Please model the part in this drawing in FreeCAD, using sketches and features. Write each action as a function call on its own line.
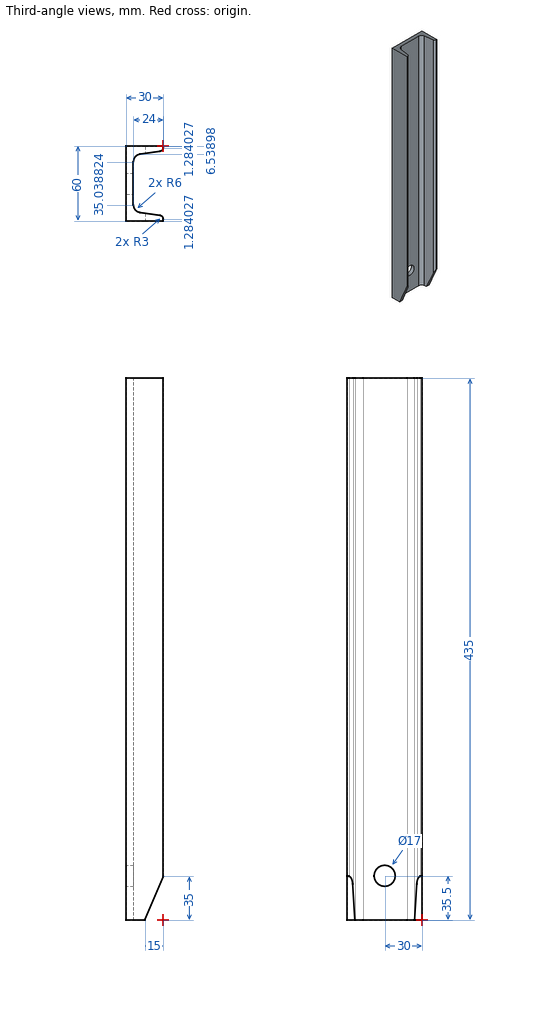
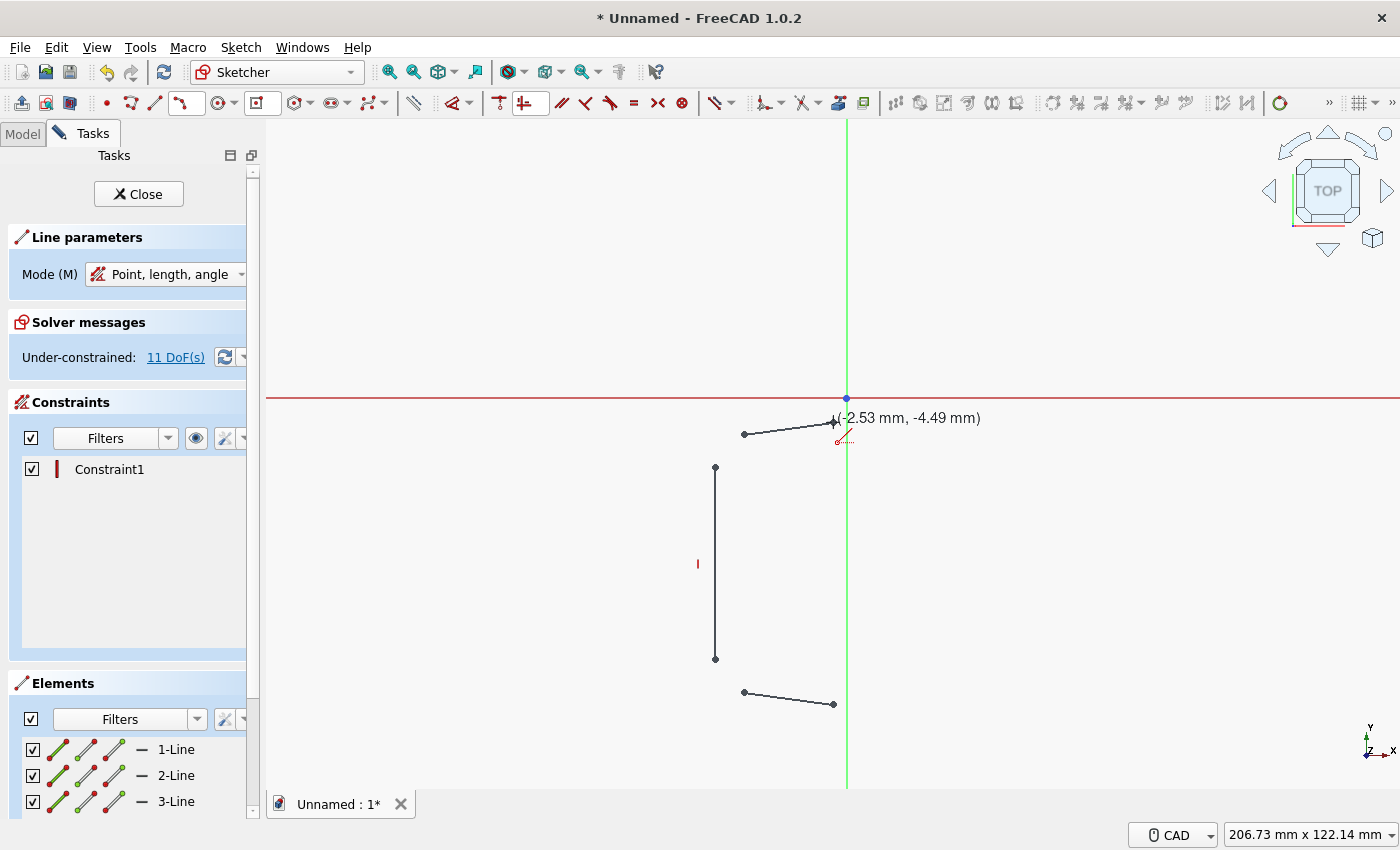
click(132, 104)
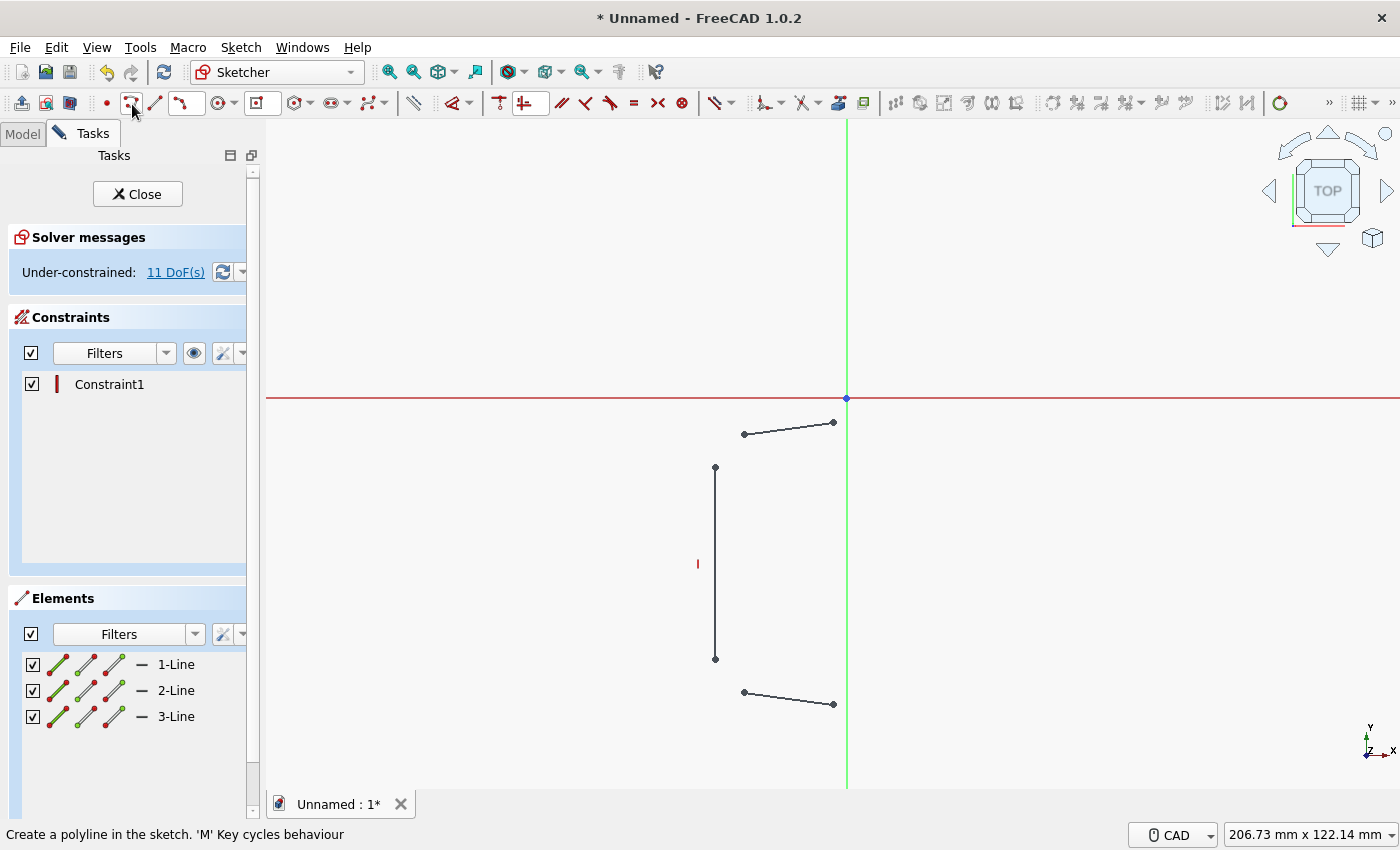
scroll(847, 405, up, 5)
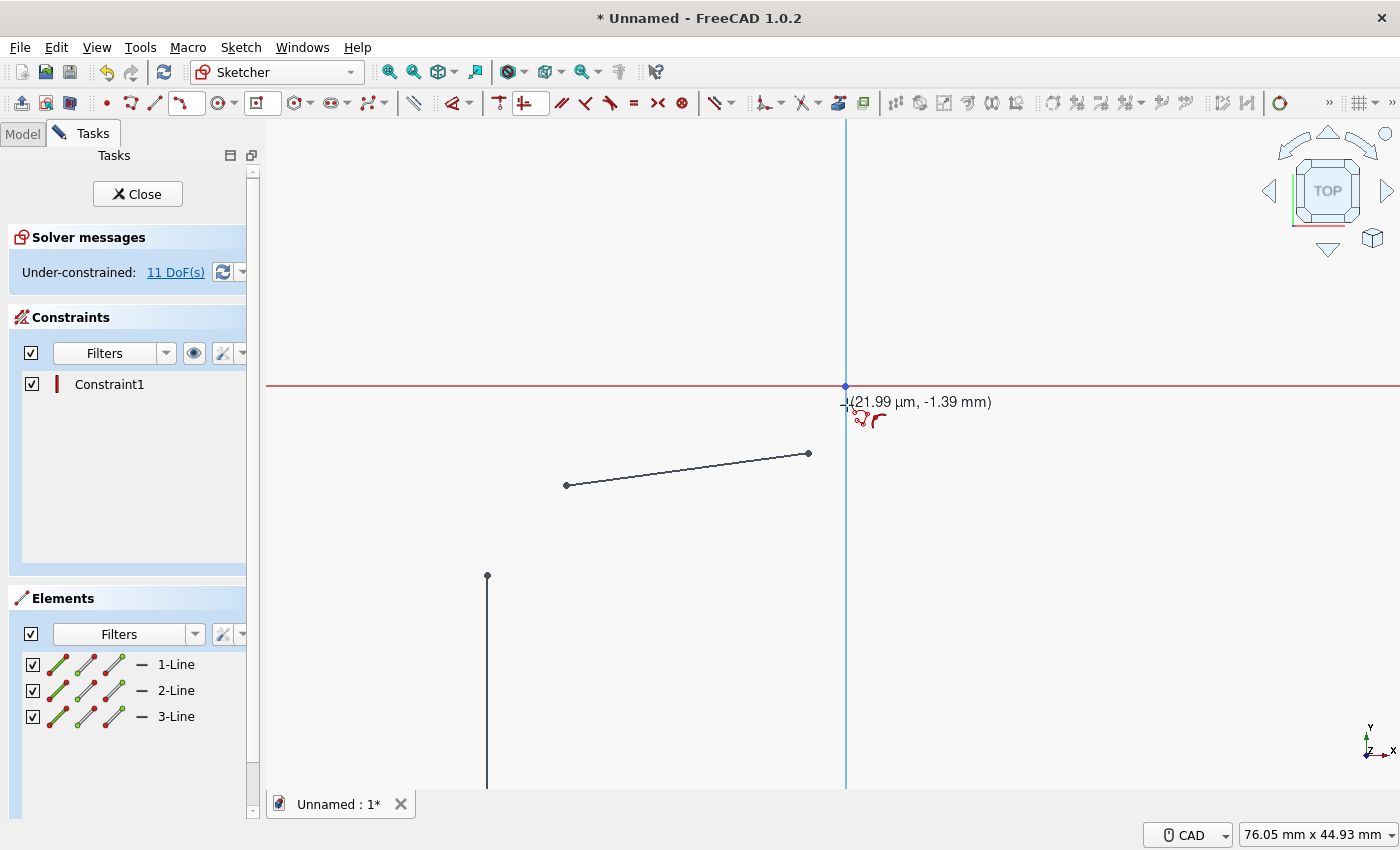
click(846, 405)
click(846, 386)
click(398, 395)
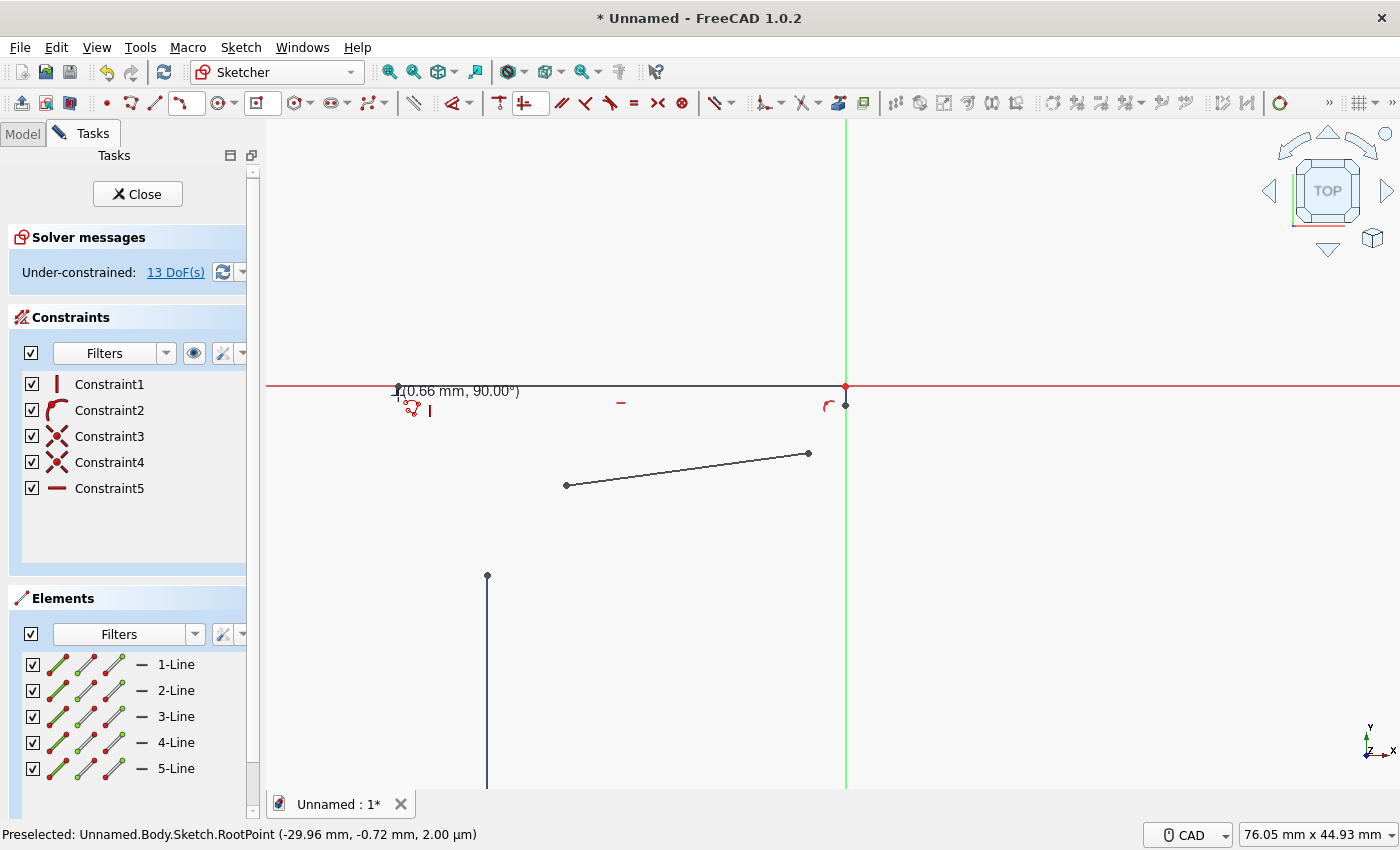
scroll(881, 147, down, 4)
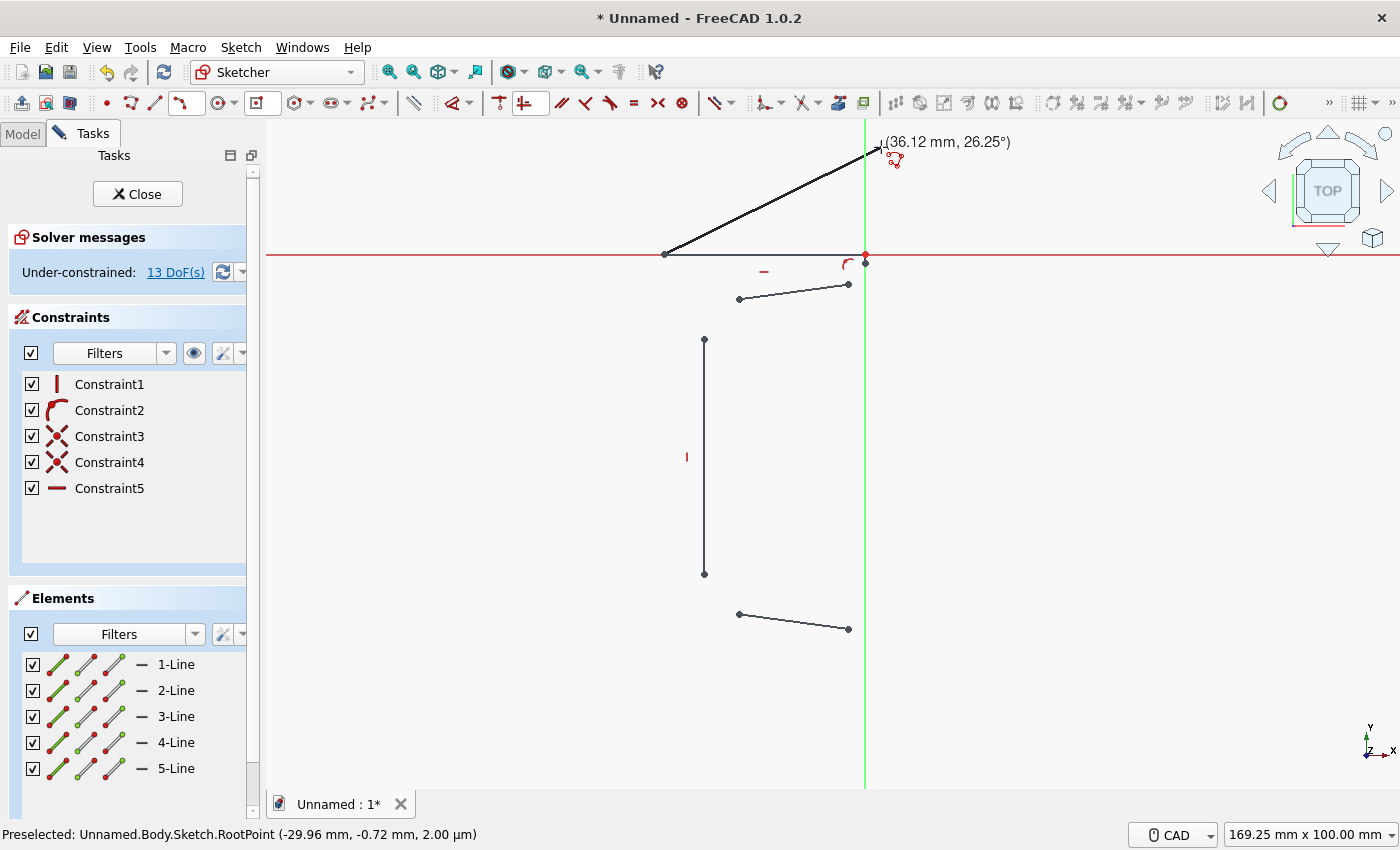
click(664, 657)
click(865, 657)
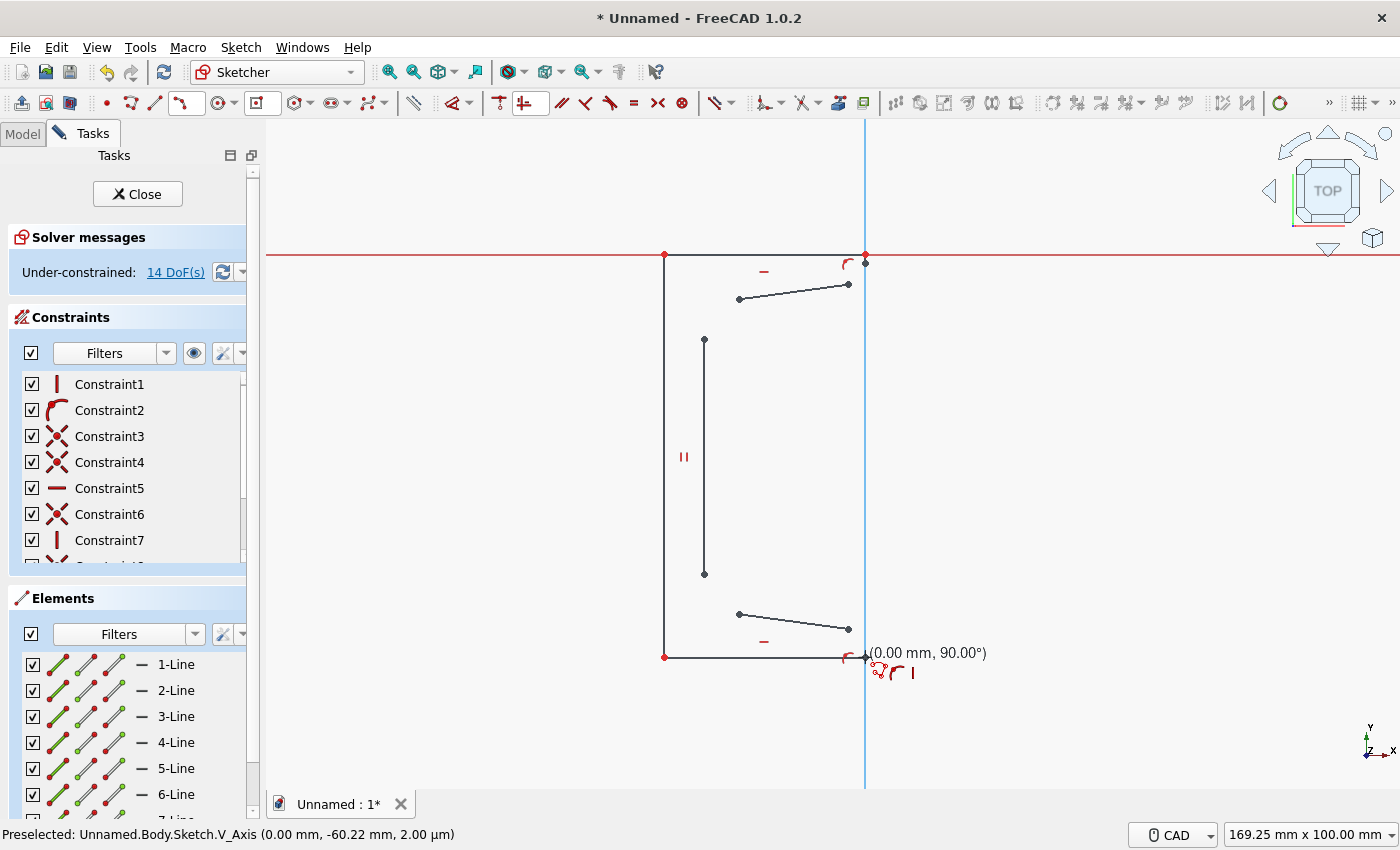
scroll(865, 648, up, 4)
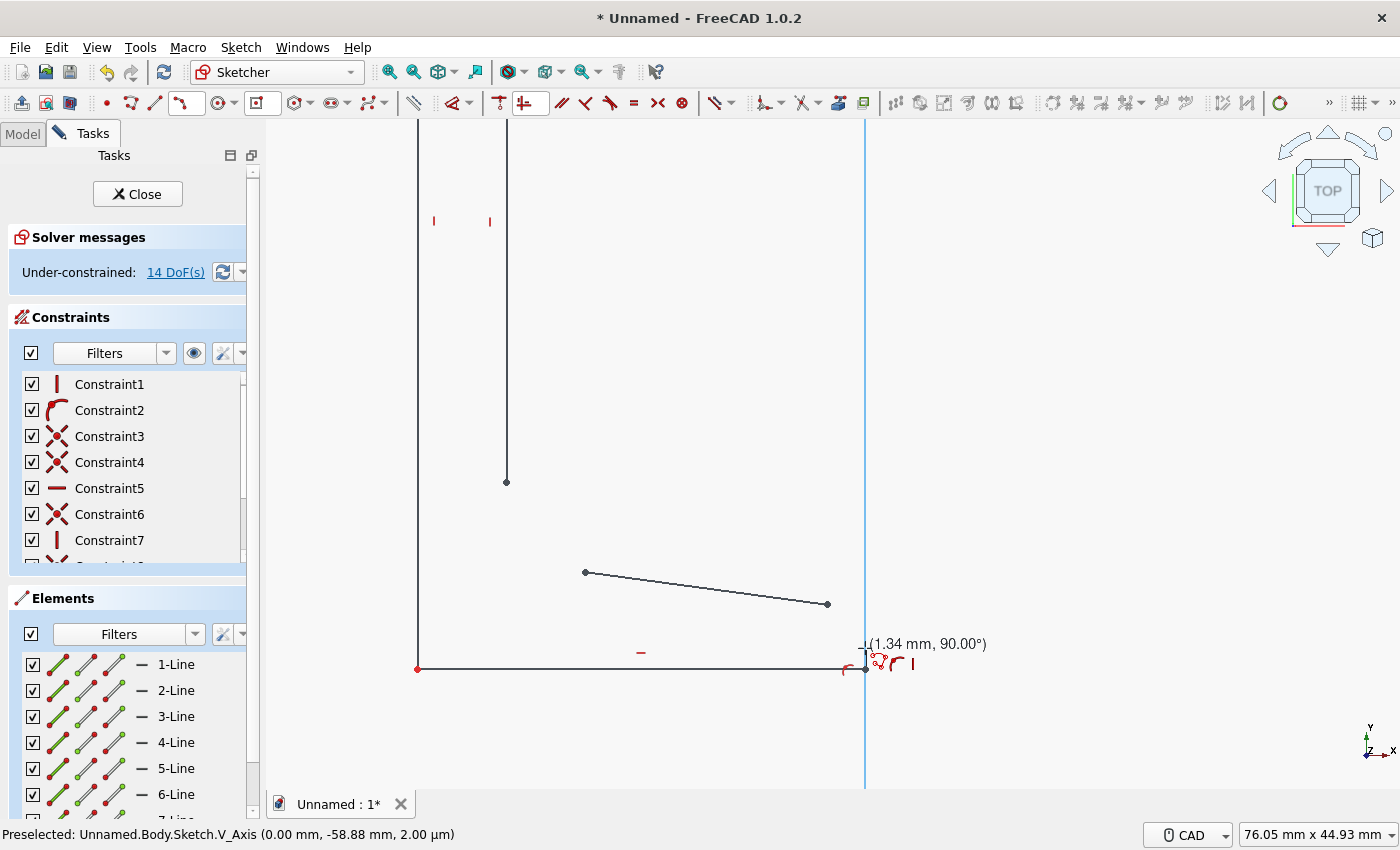
click(856, 647)
right_click(856, 647)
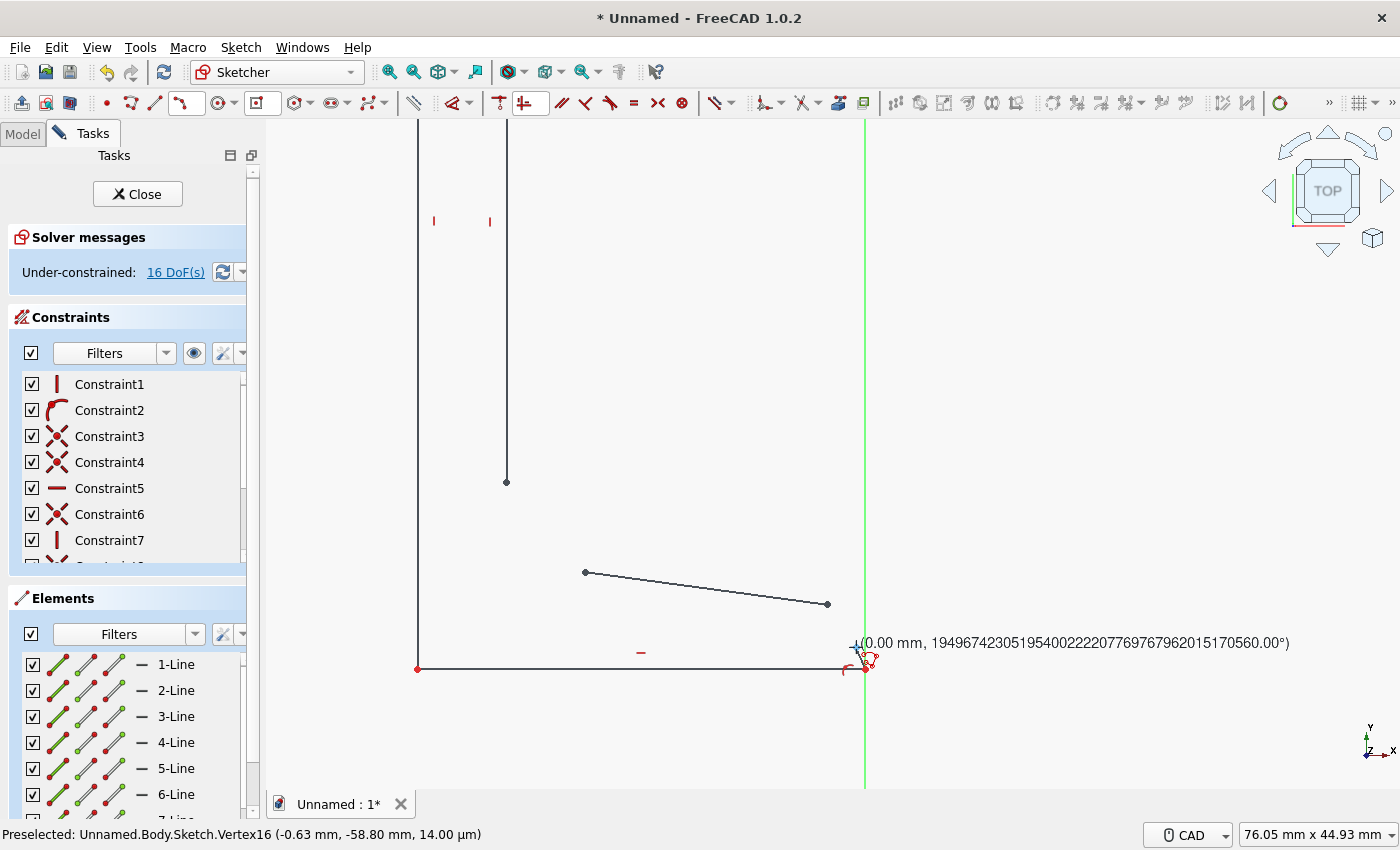
click(180, 104)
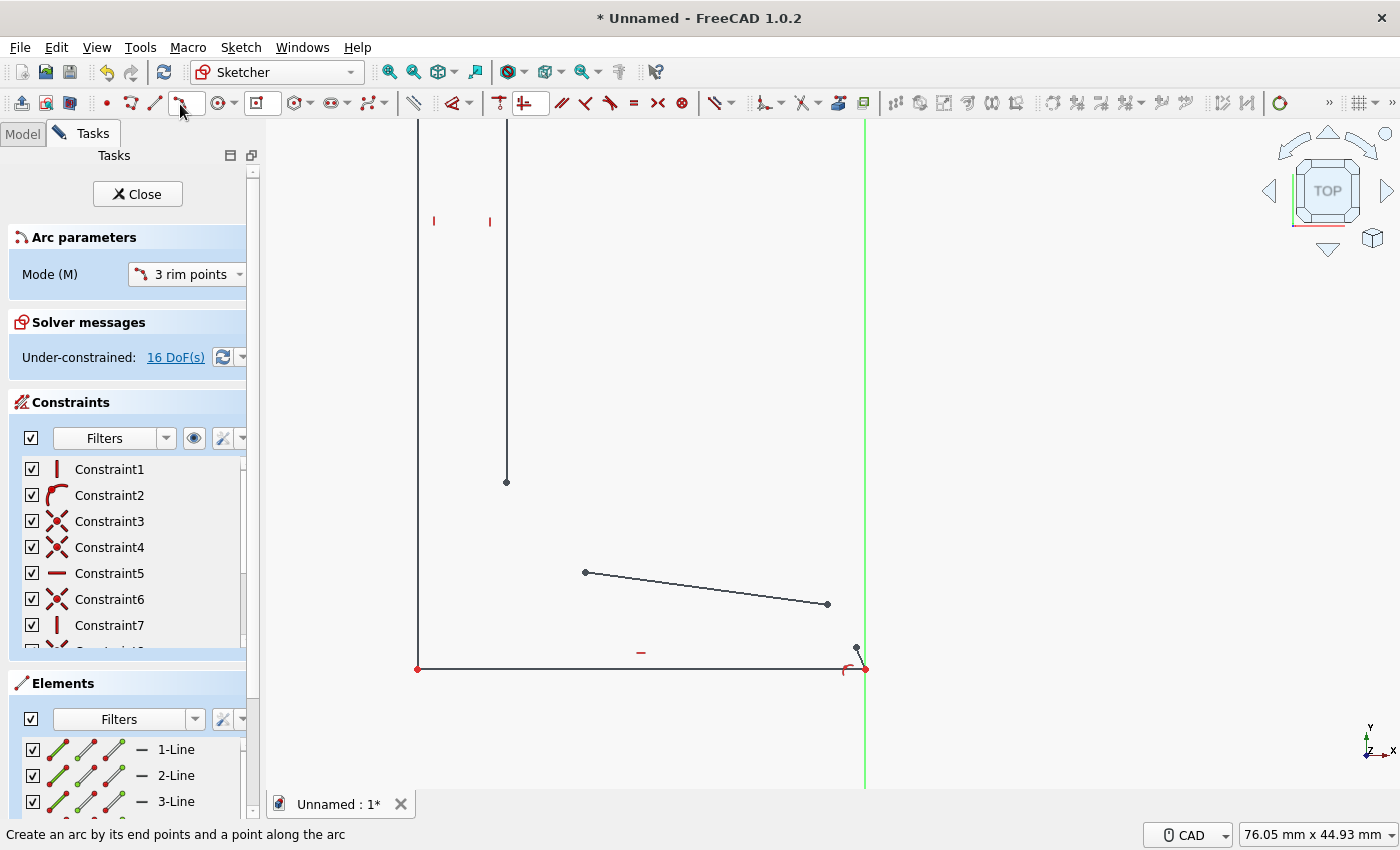
click(586, 572)
click(507, 483)
click(529, 539)